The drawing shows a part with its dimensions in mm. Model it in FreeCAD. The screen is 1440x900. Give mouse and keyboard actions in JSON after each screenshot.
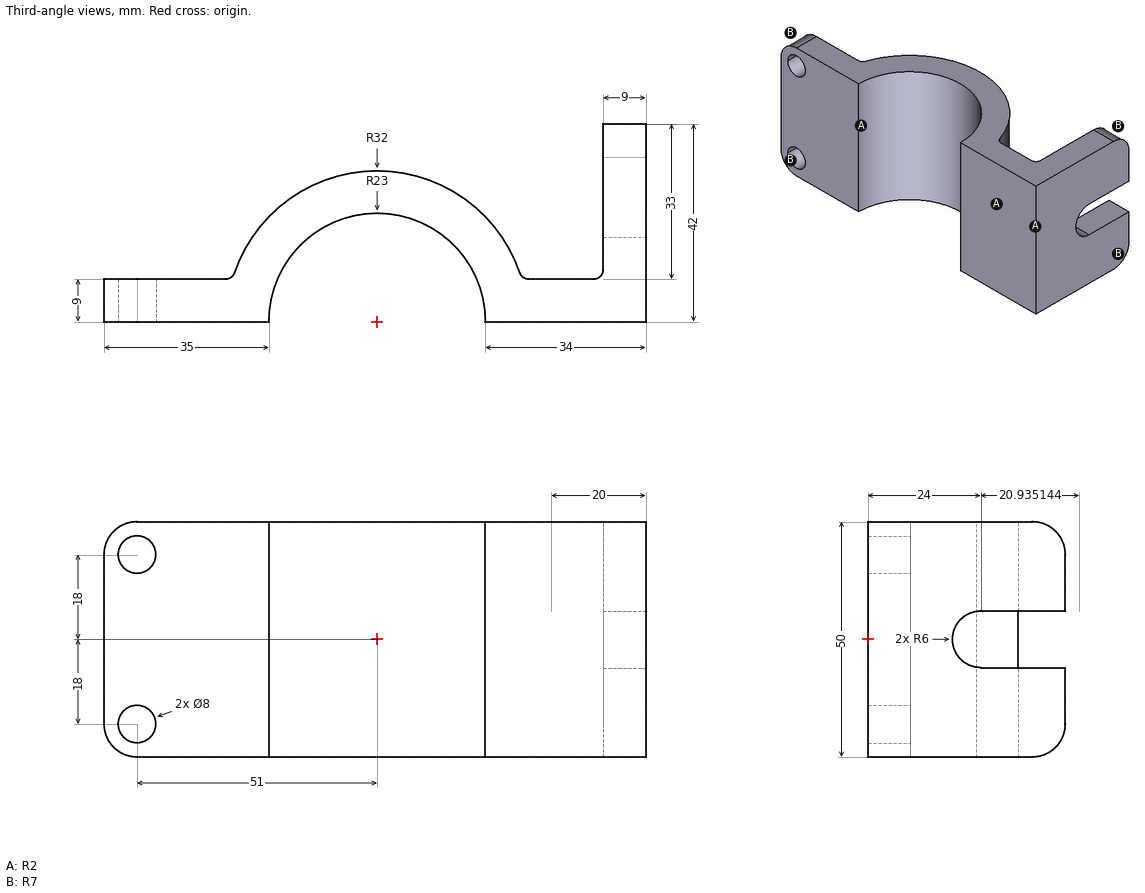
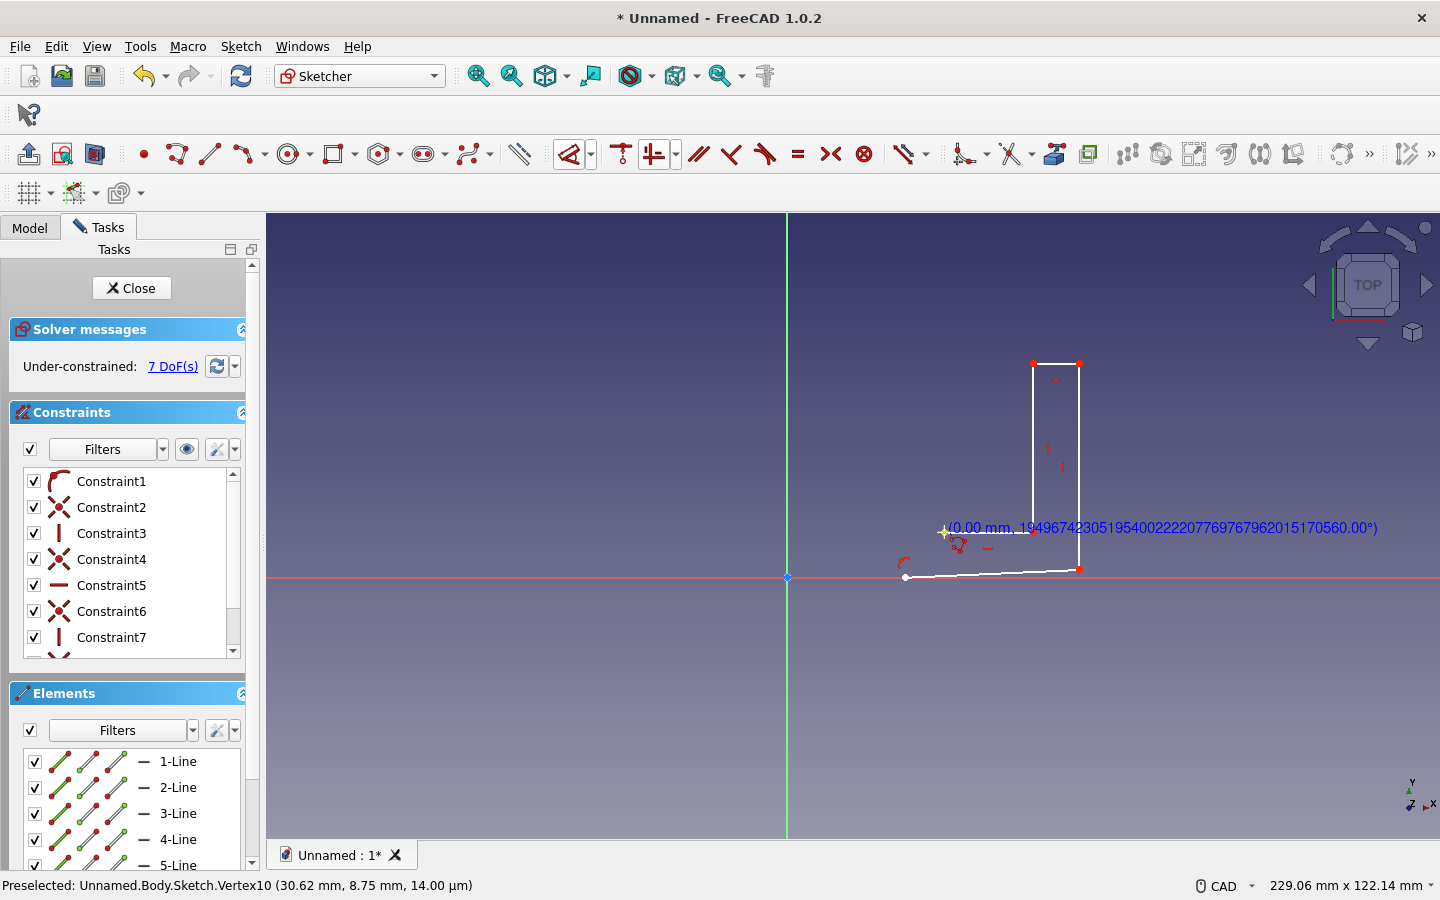
{"action": "left_click", "coordinate": [630, 532]}
{"action": "left_click", "coordinate": [490, 532]}
{"action": "left_click", "coordinate": [490, 578]}
{"action": "left_click", "coordinate": [669, 569]}
{"action": "right_click", "coordinate": [669, 569]}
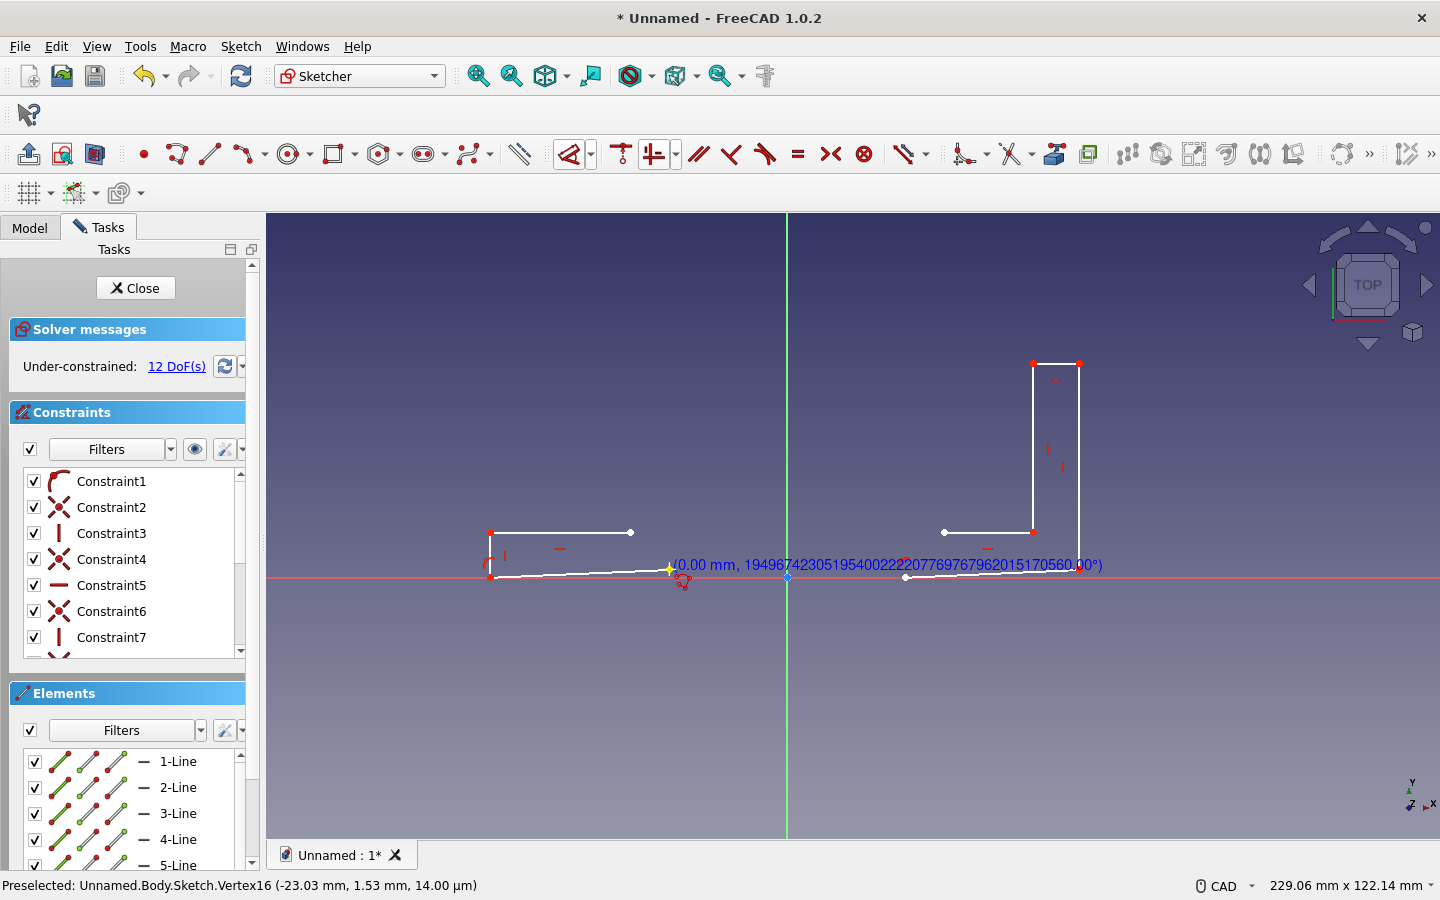
{"action": "left_click", "coordinate": [242, 154]}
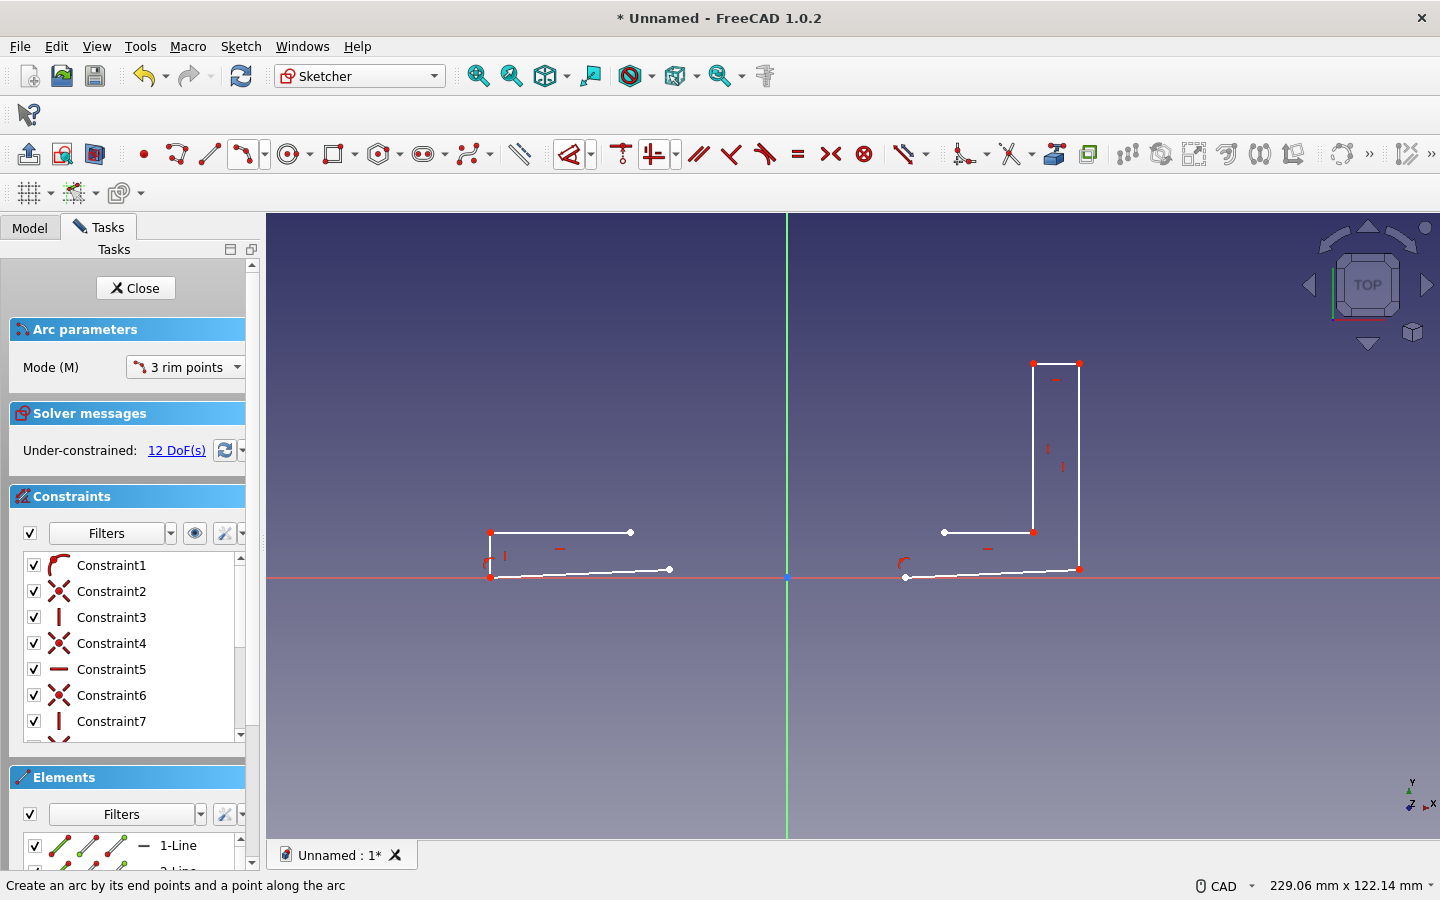
{"action": "left_click", "coordinate": [944, 533]}
{"action": "left_click", "coordinate": [630, 533]}
{"action": "left_click", "coordinate": [829, 419]}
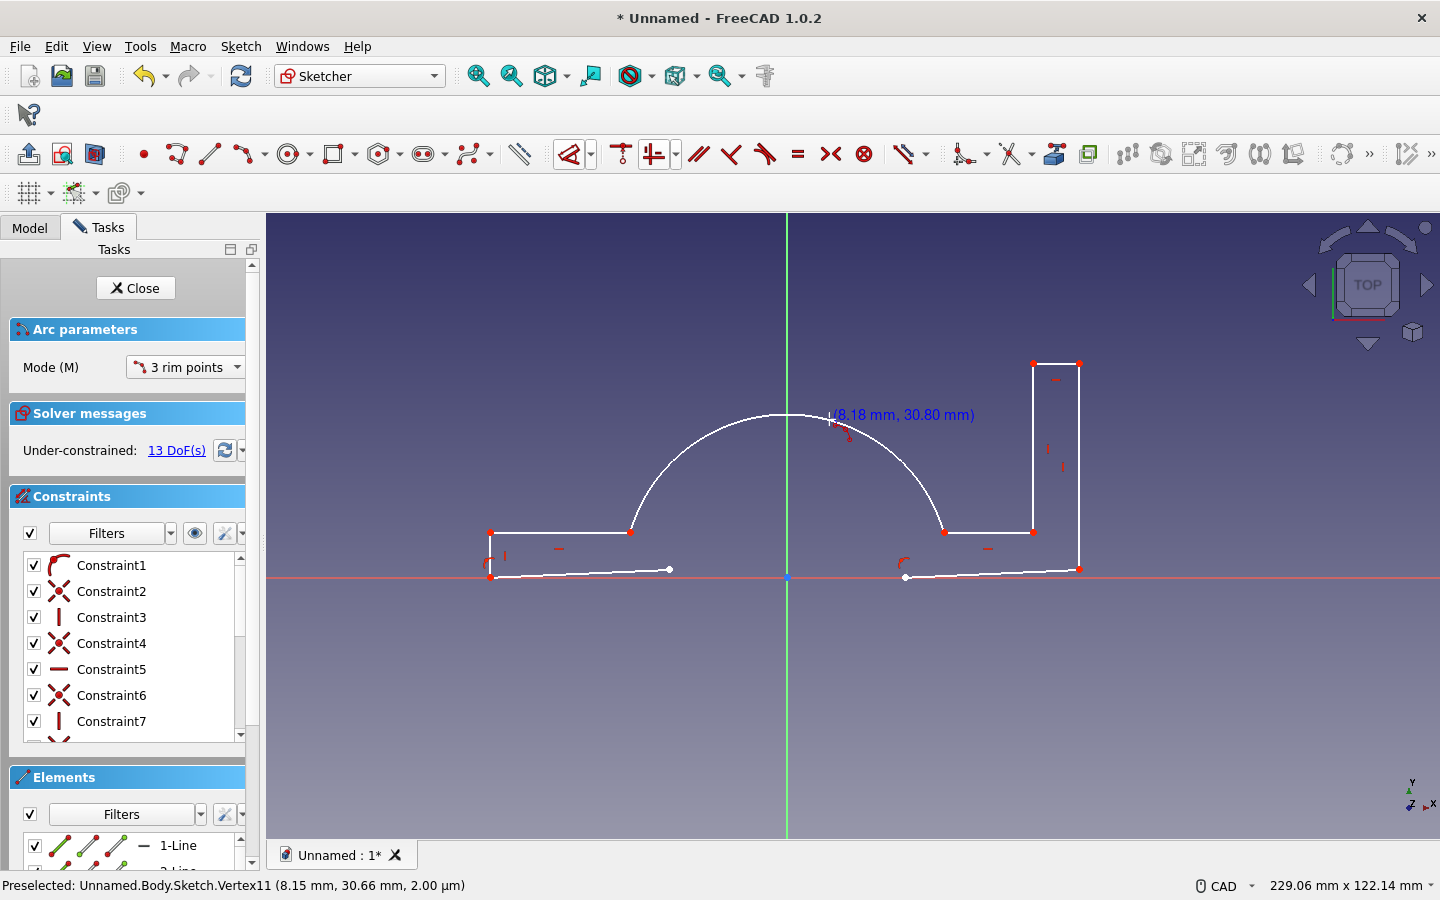
{"action": "left_click", "coordinate": [669, 570]}
{"action": "left_click", "coordinate": [905, 578]}
{"action": "left_click", "coordinate": [823, 466]}
{"action": "key", "text": "Escape"}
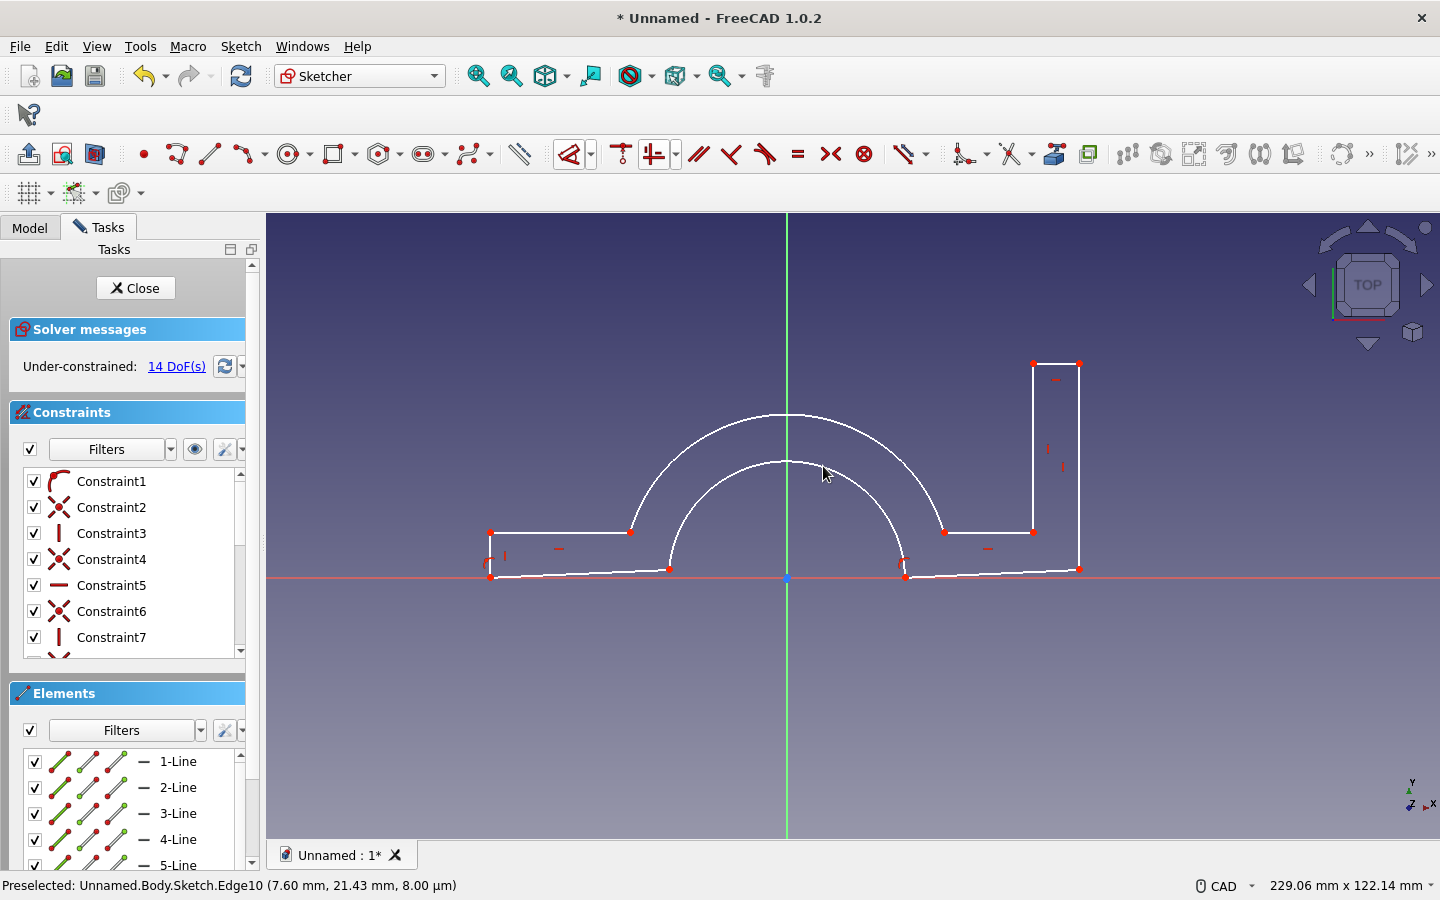
{"action": "left_click", "coordinate": [957, 575]}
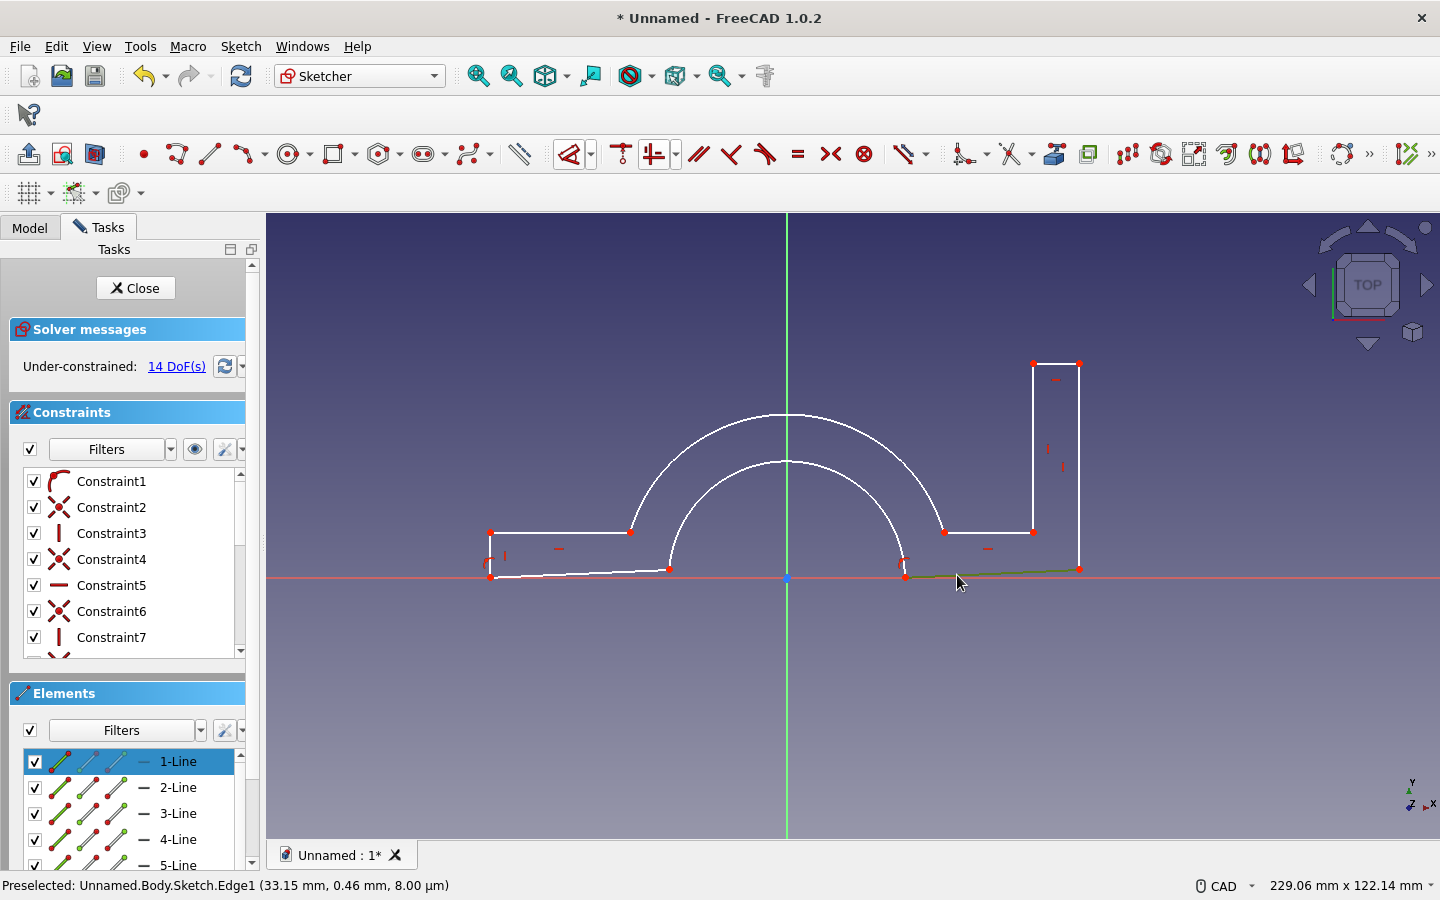
{"action": "key", "text": "h"}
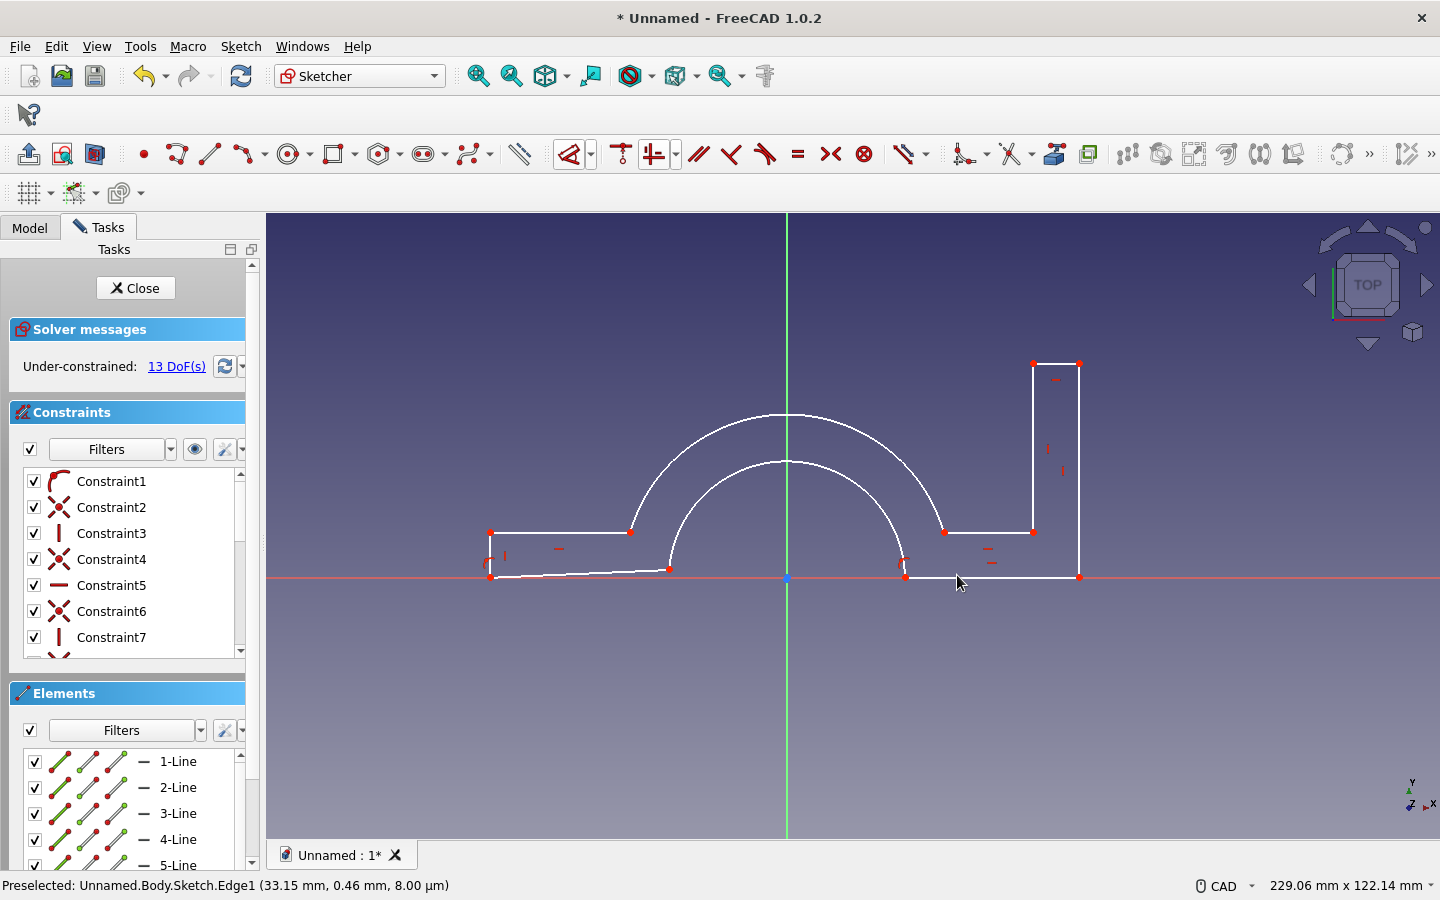
{"action": "left_click", "coordinate": [544, 575]}